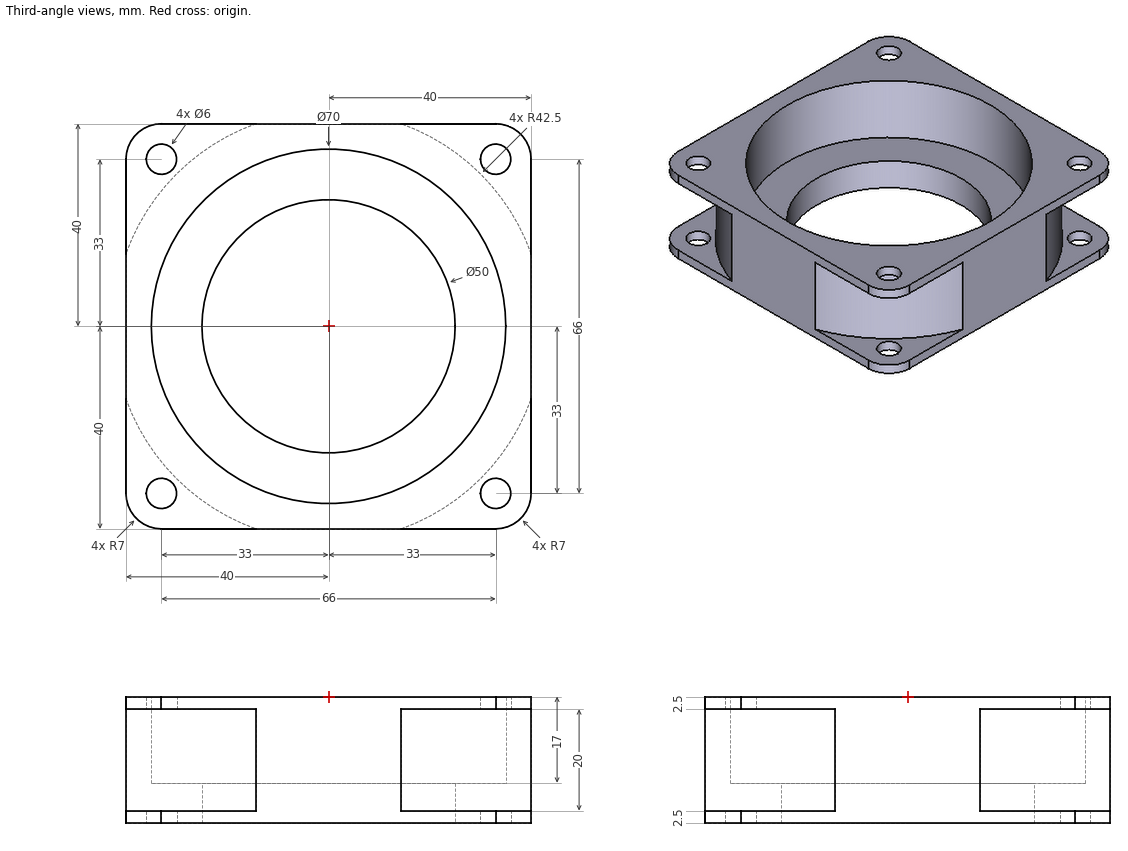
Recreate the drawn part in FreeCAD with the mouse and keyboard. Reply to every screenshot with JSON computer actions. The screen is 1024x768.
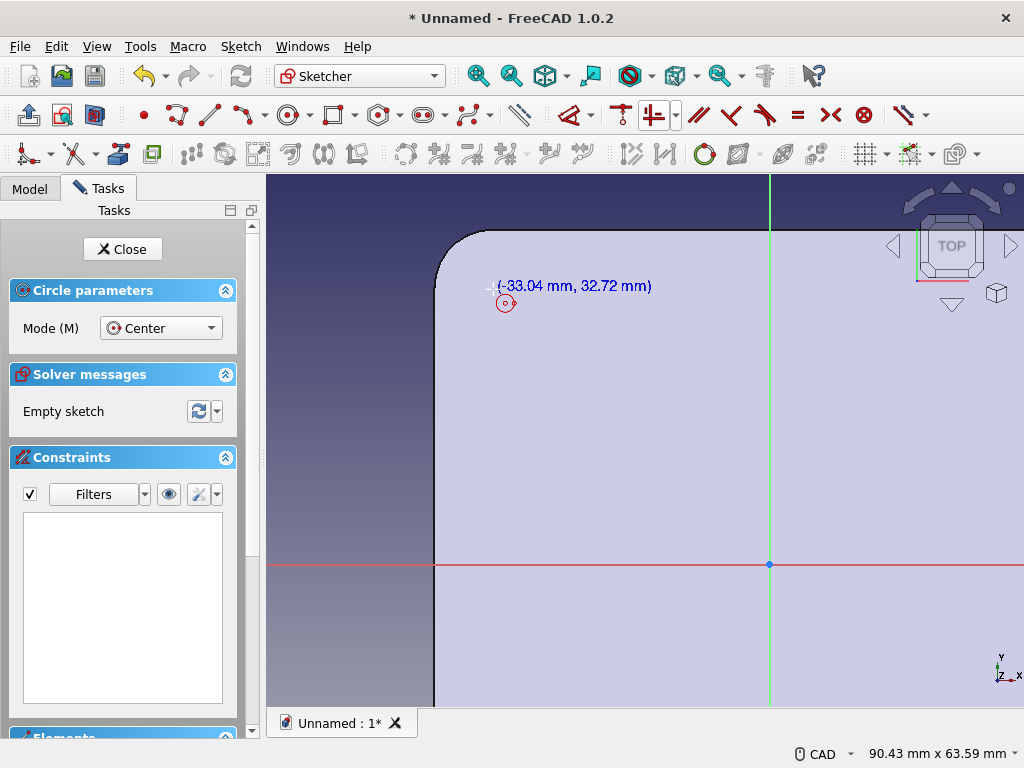
{"action": "left_click", "coordinate": [493, 288]}
{"action": "mouse_move", "coordinate": [511, 270]}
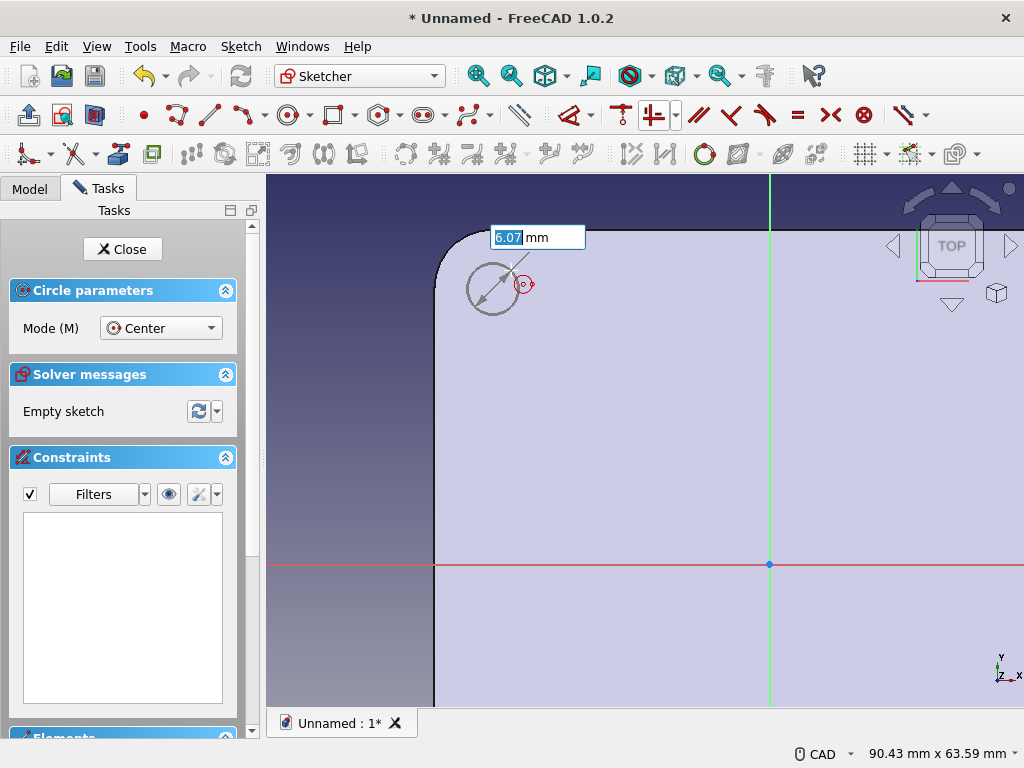
{"action": "type", "text": "6"}
{"action": "key", "text": "Return"}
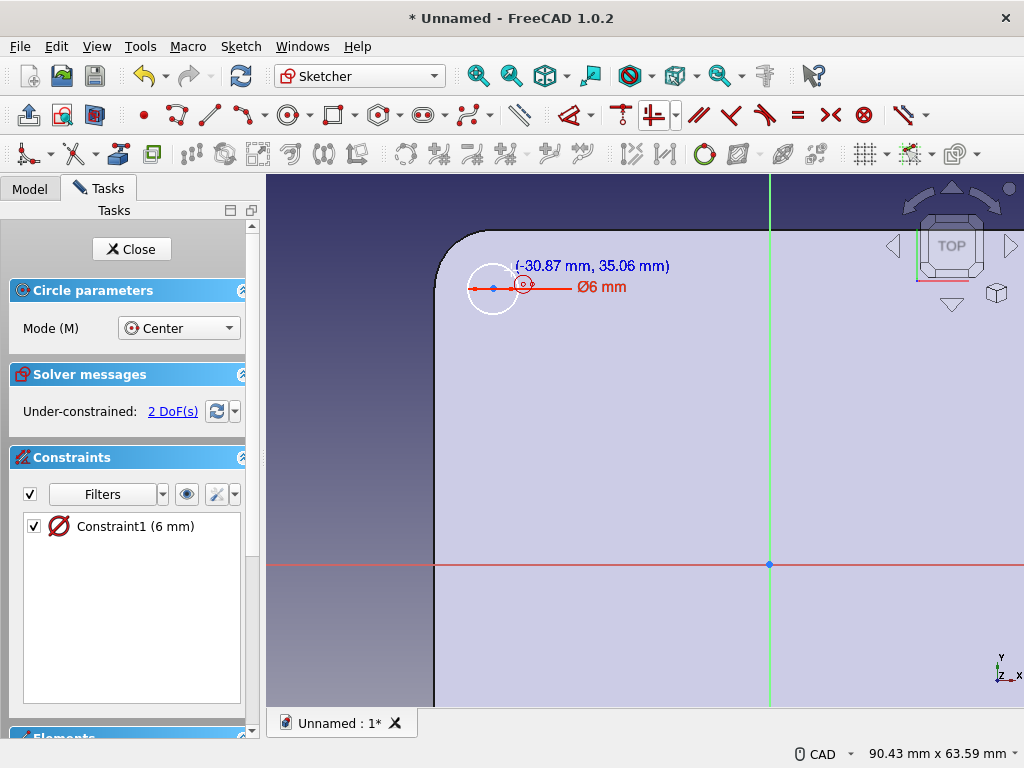
{"action": "scroll", "coordinate": [341, 289], "scroll_direction": "down", "scroll_amount": 3}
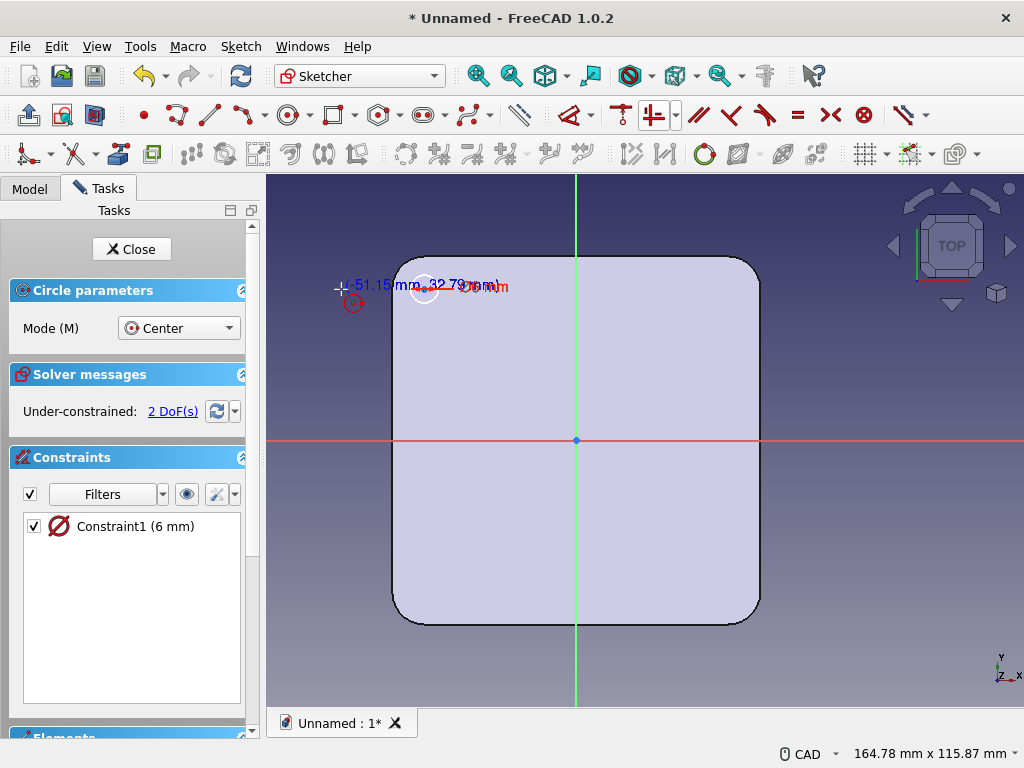
{"action": "scroll", "coordinate": [728, 289], "scroll_direction": "up", "scroll_amount": 3}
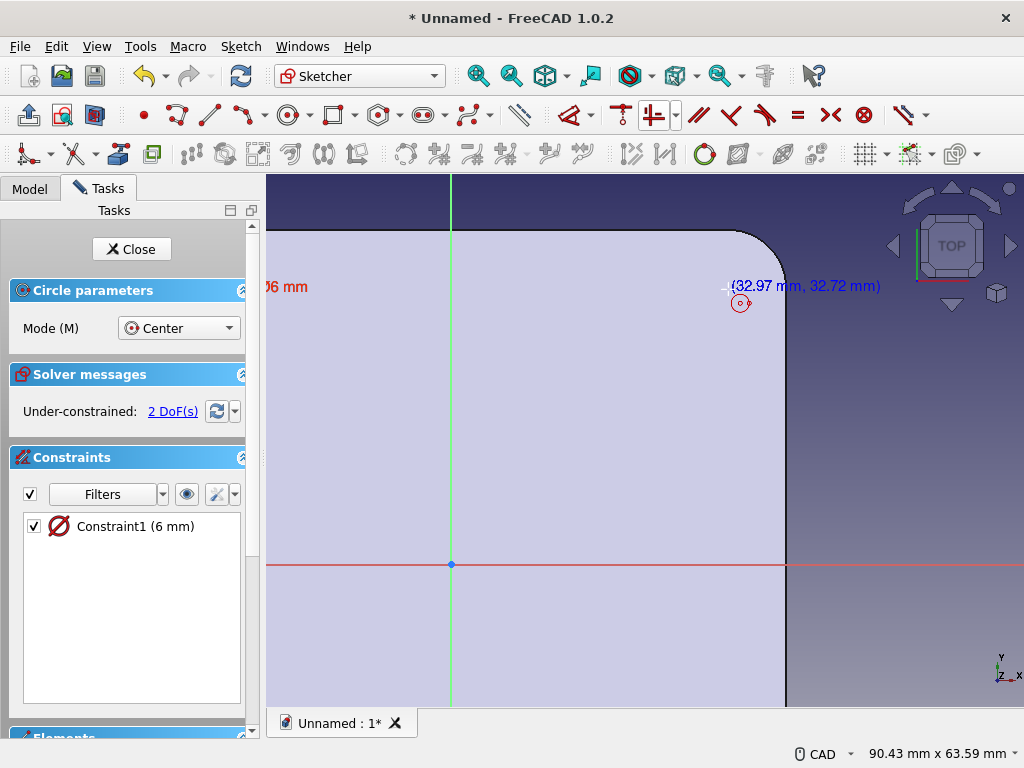
{"action": "left_click", "coordinate": [728, 288]}
{"action": "mouse_move", "coordinate": [746, 270]}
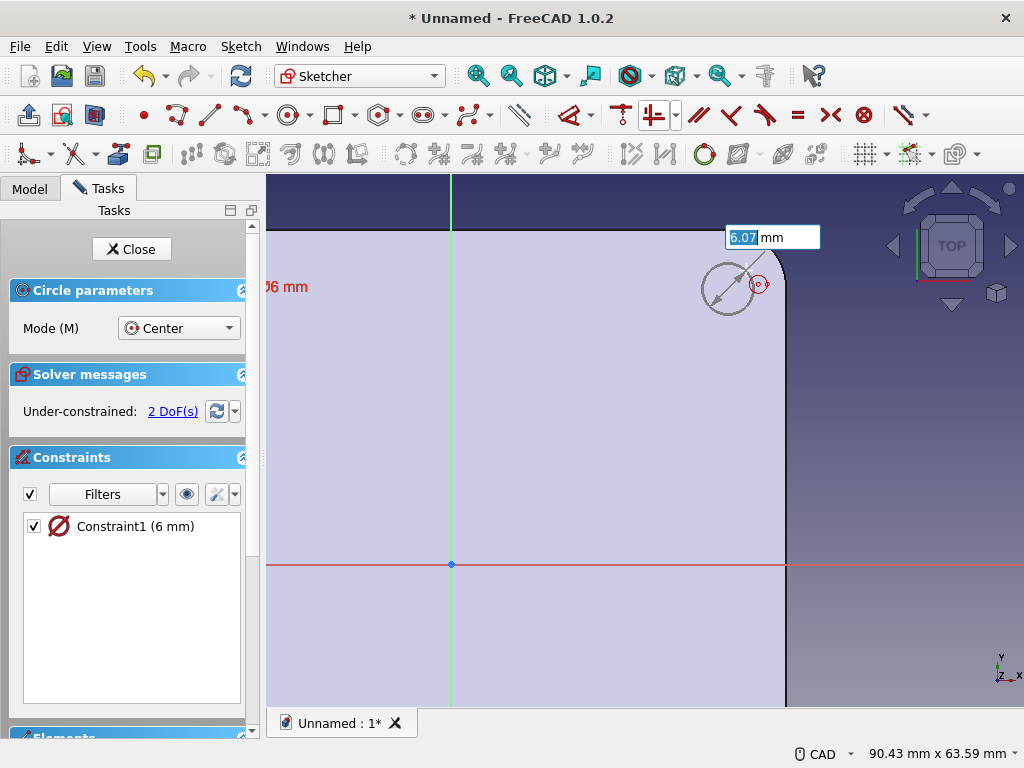
{"action": "type", "text": "6"}
{"action": "key", "text": "Return"}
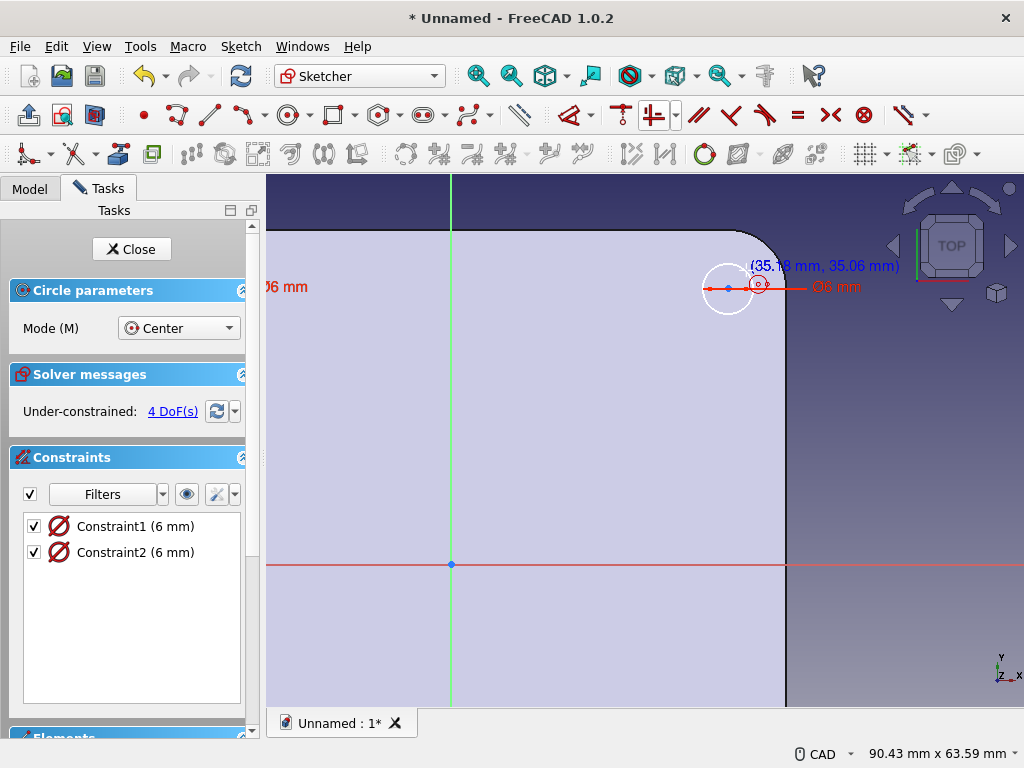
{"action": "scroll", "coordinate": [729, 289], "scroll_direction": "down", "scroll_amount": 3}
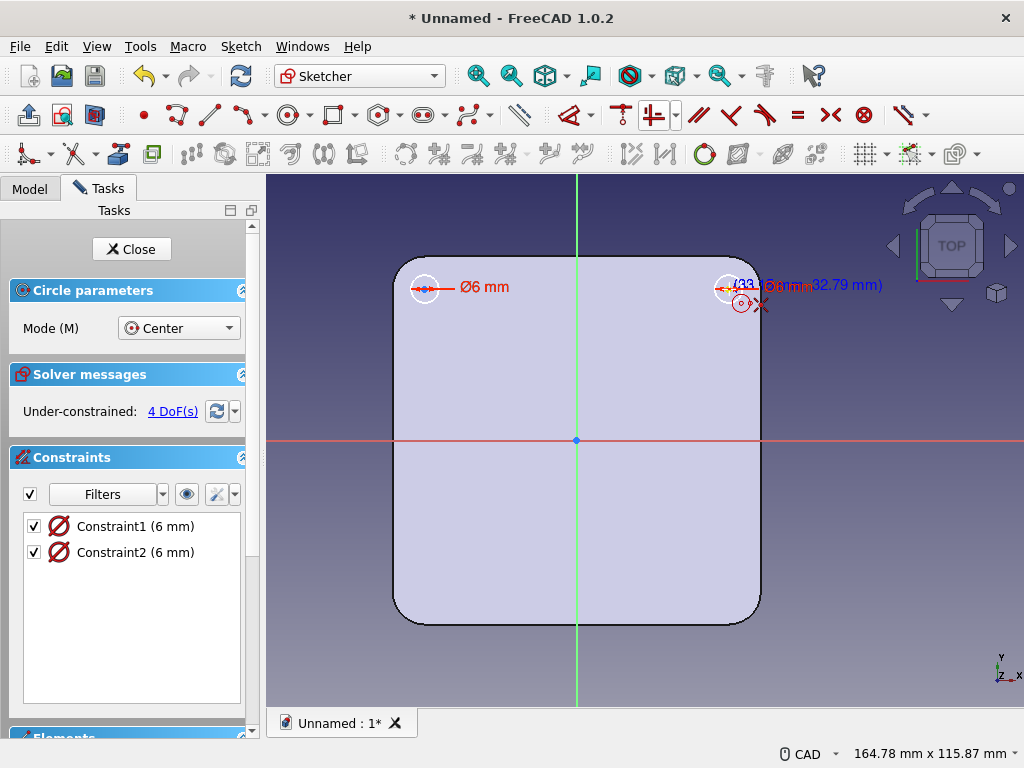
{"action": "scroll", "coordinate": [729, 592], "scroll_direction": "up", "scroll_amount": 3}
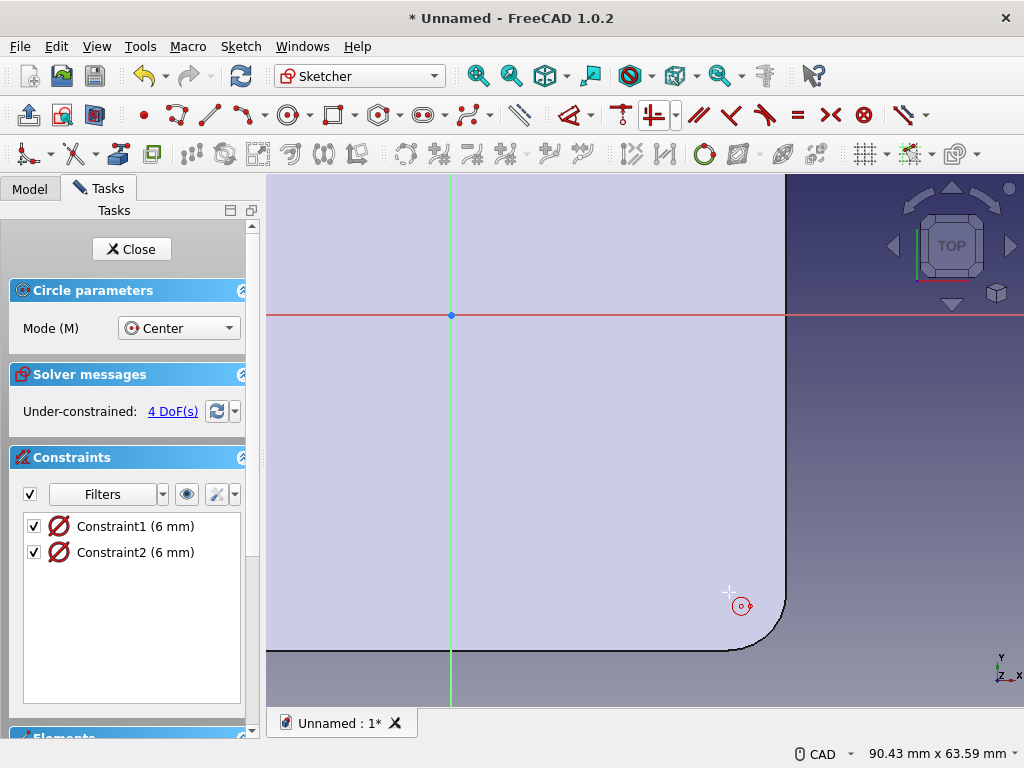
{"action": "left_click", "coordinate": [728, 592]}
{"action": "mouse_move", "coordinate": [746, 574]}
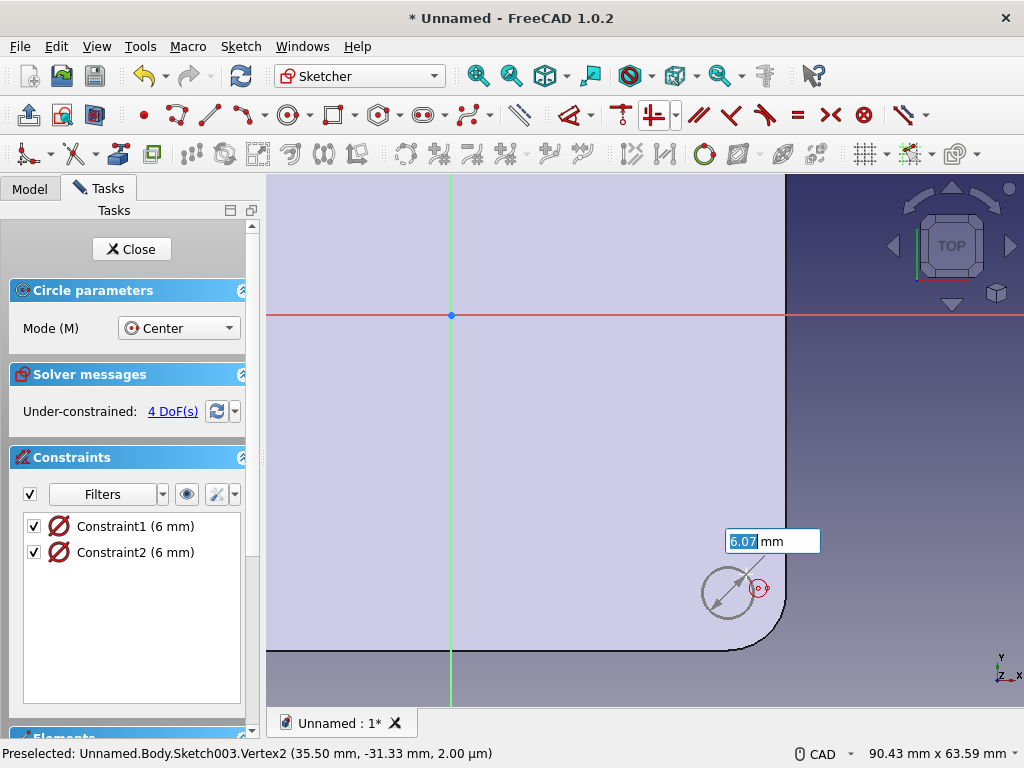
{"action": "type", "text": "6"}
{"action": "key", "text": "Return"}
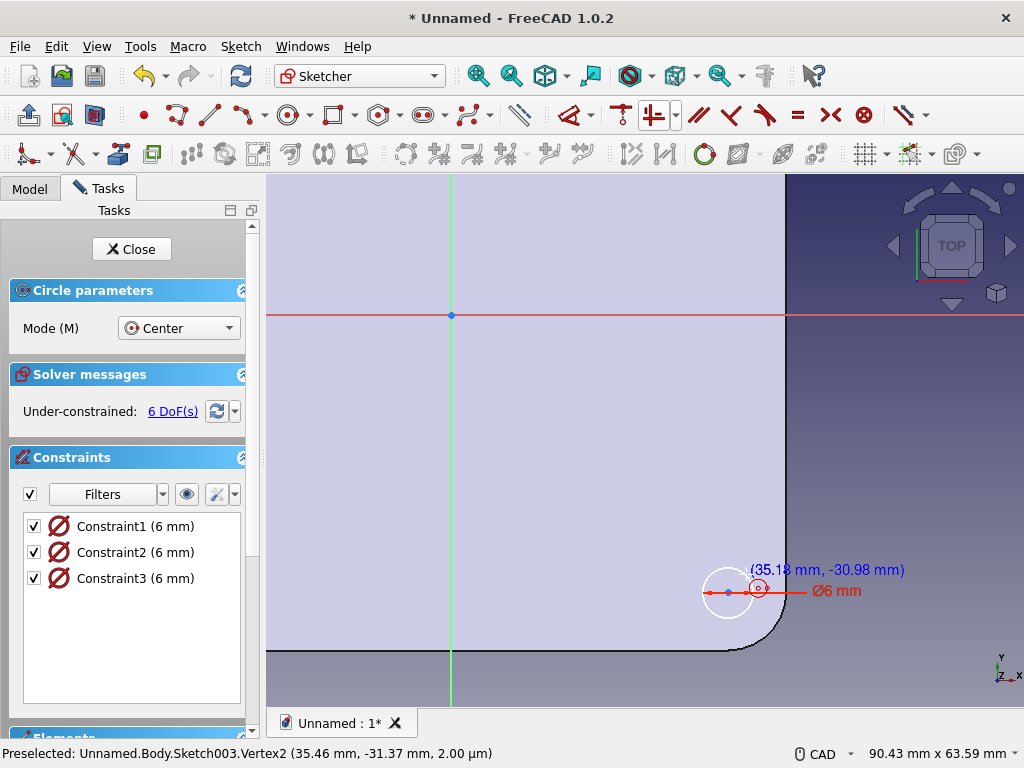
{"action": "scroll", "coordinate": [729, 593], "scroll_direction": "down", "scroll_amount": 3}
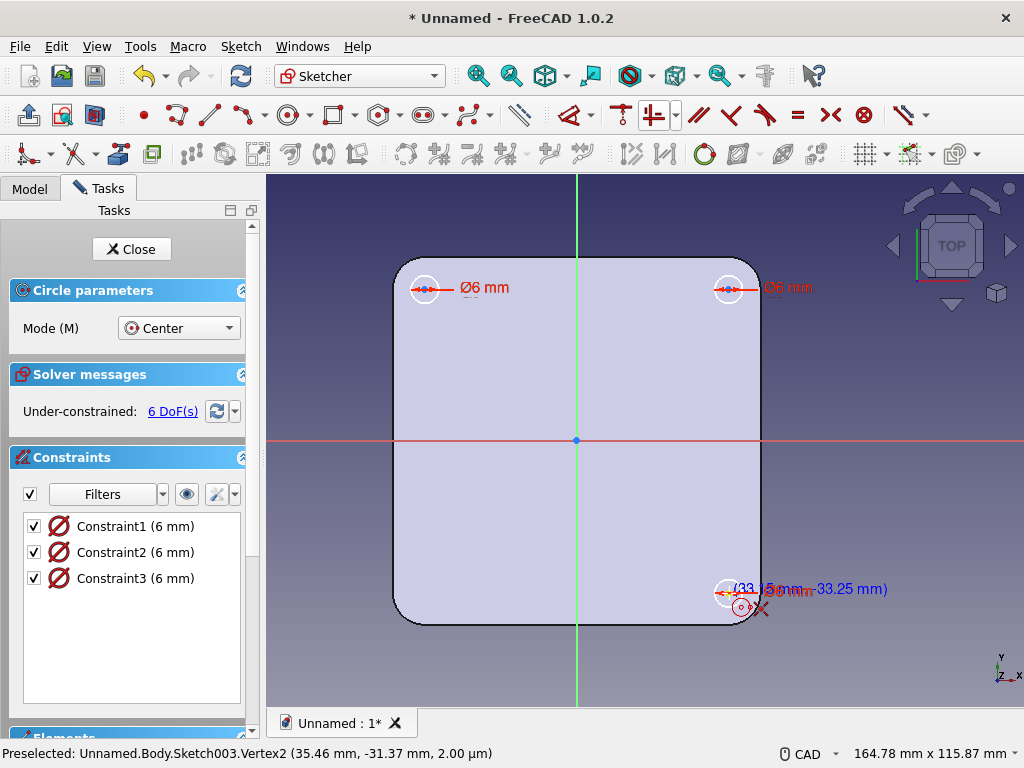
{"action": "scroll", "coordinate": [425, 593], "scroll_direction": "up", "scroll_amount": 3}